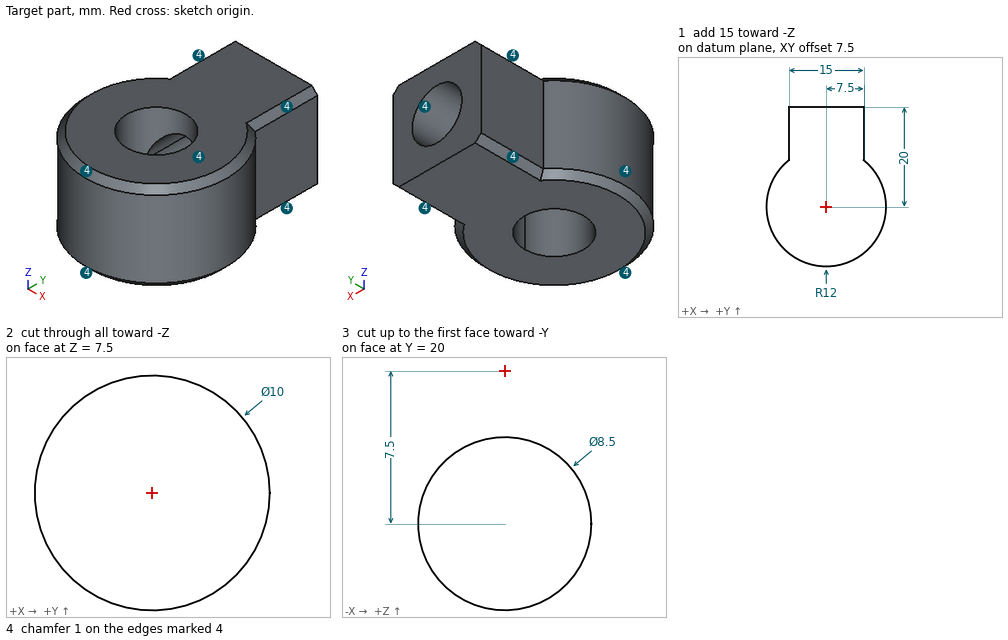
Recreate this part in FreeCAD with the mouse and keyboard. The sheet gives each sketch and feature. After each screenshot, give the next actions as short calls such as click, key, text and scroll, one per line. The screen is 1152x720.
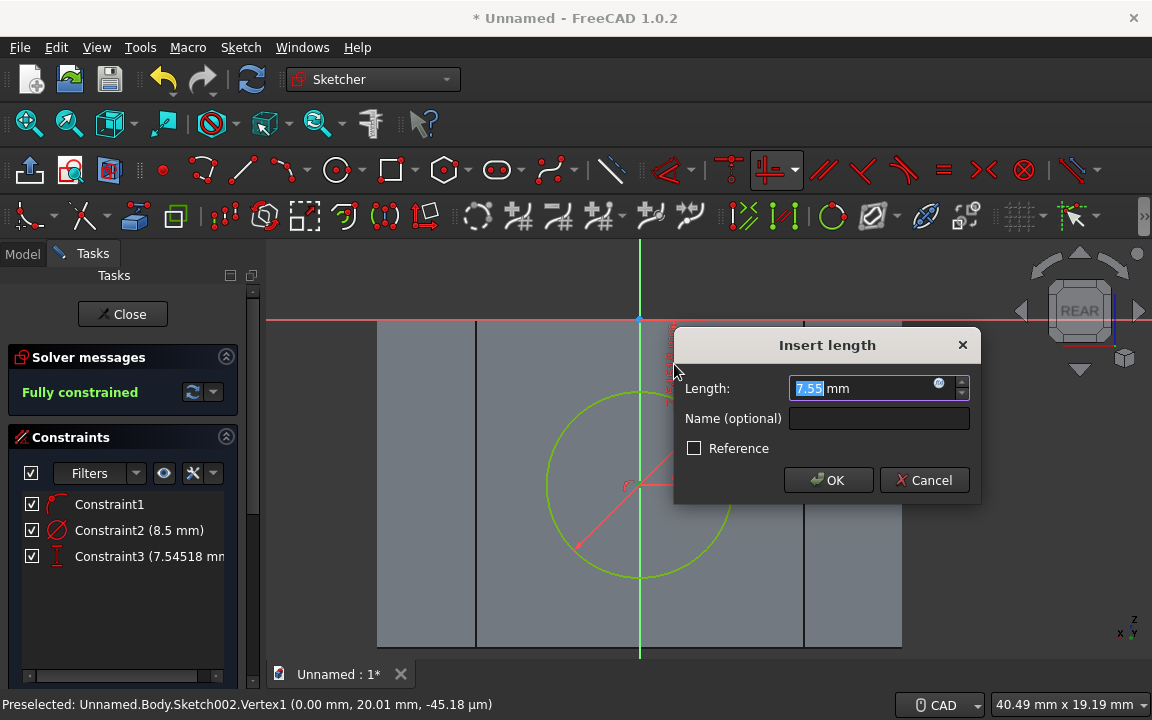
text(7.5)
key(Return)
key(Escape)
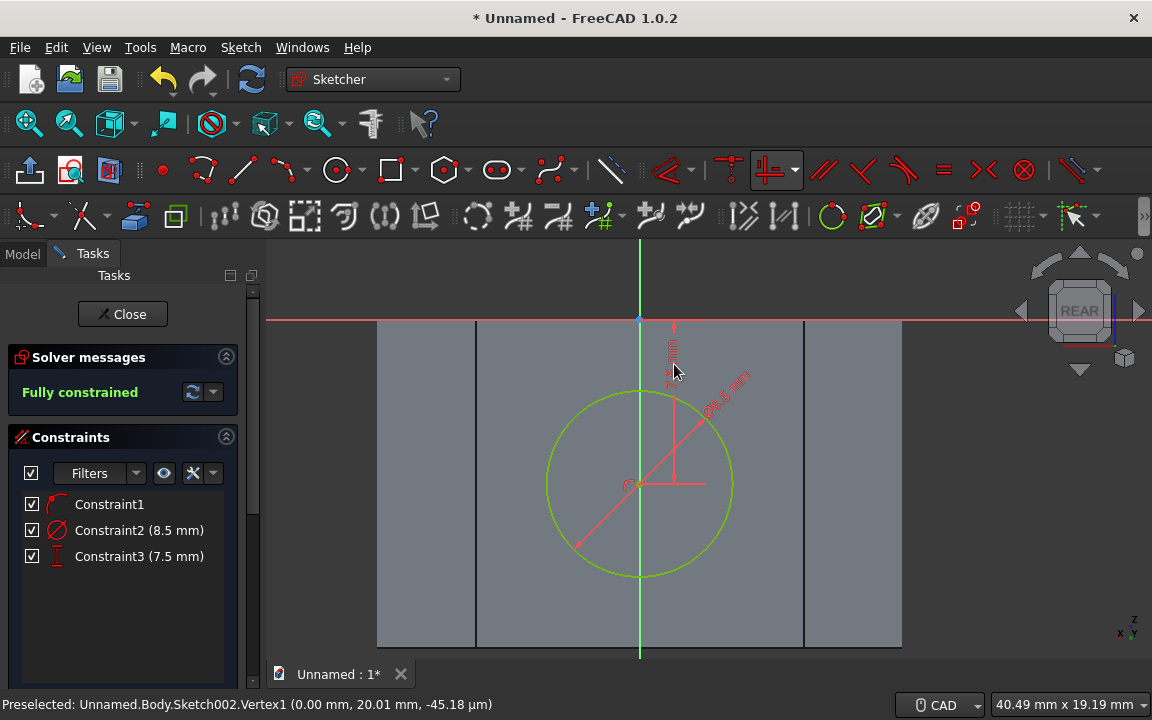
click(123, 314)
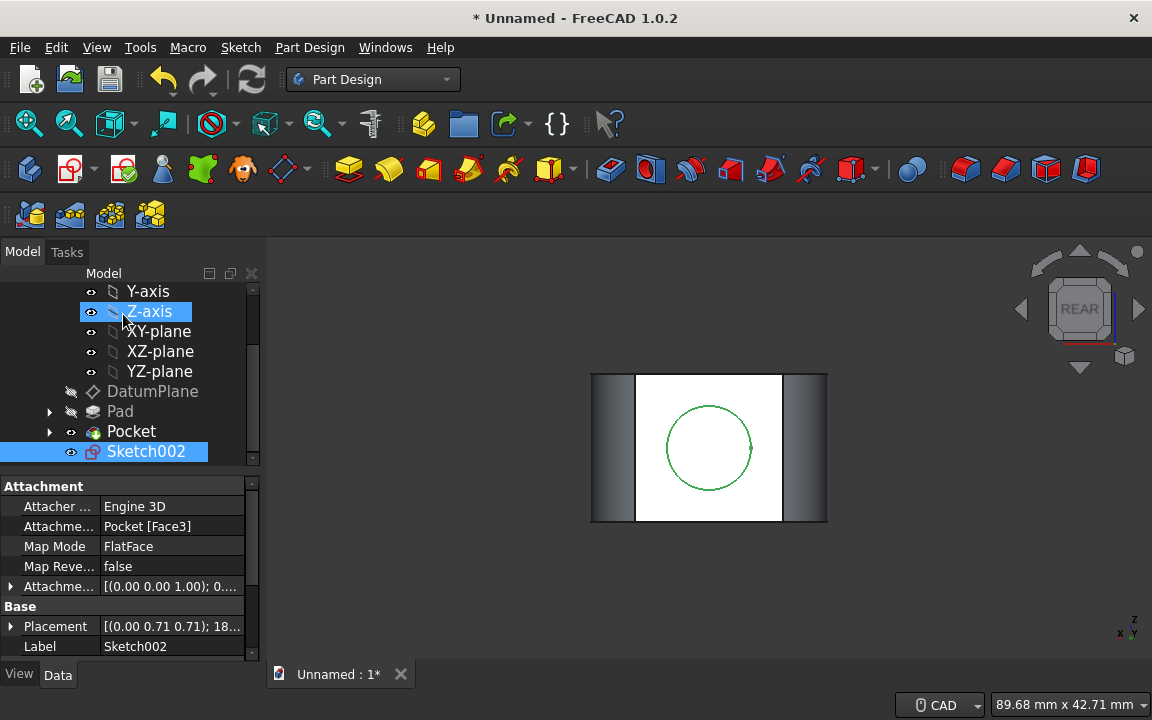
click(612, 170)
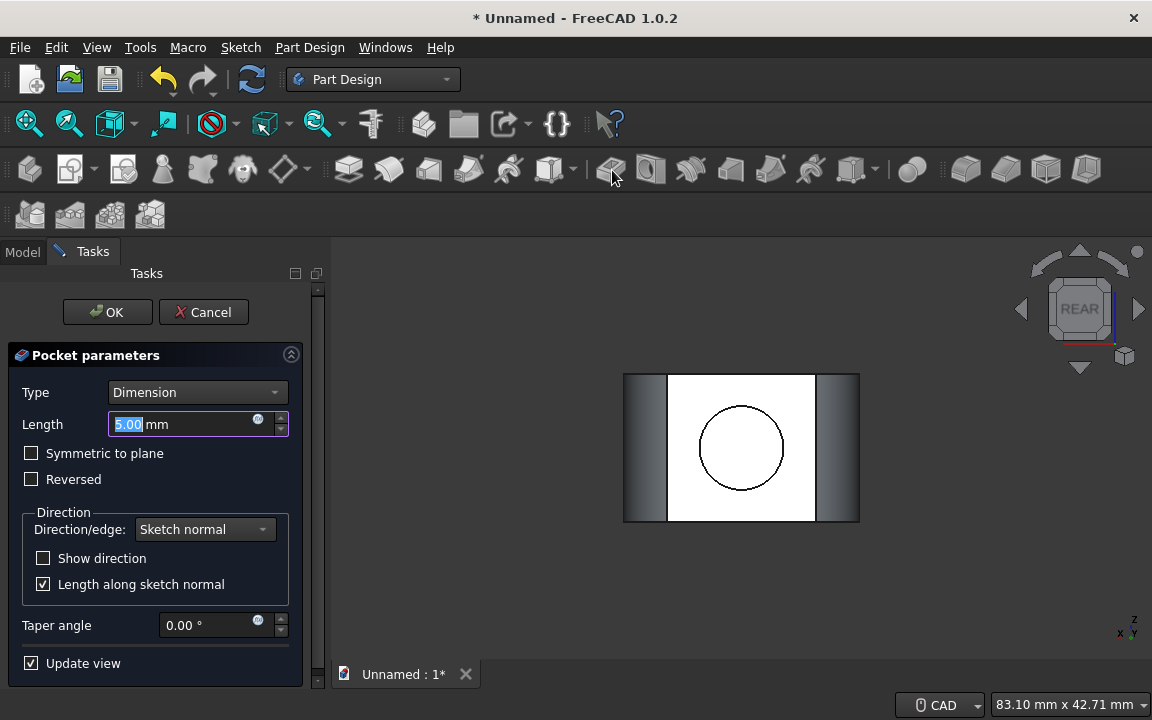
click(198, 392)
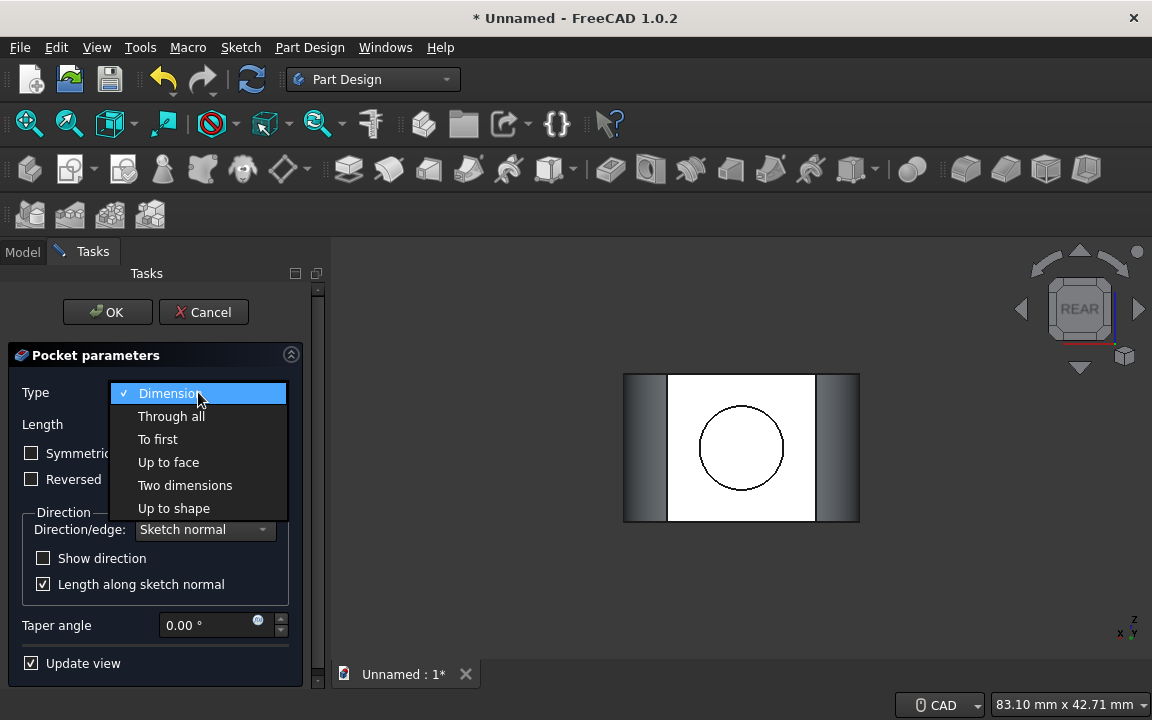
click(198, 440)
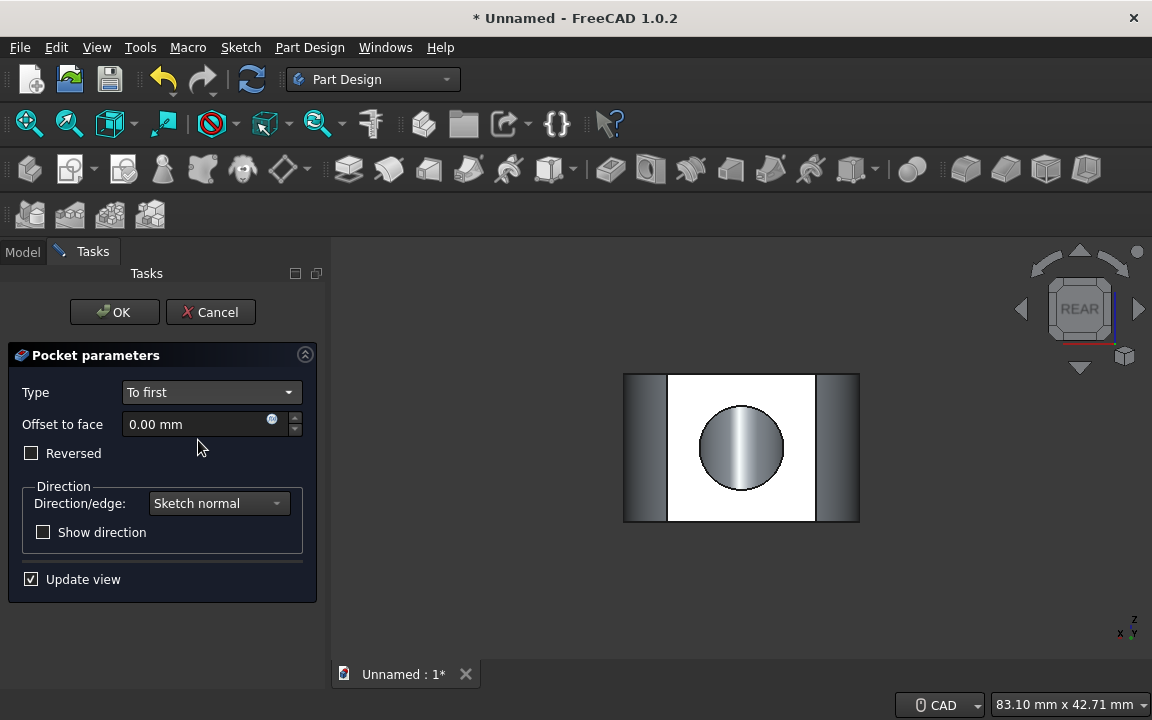
click(115, 312)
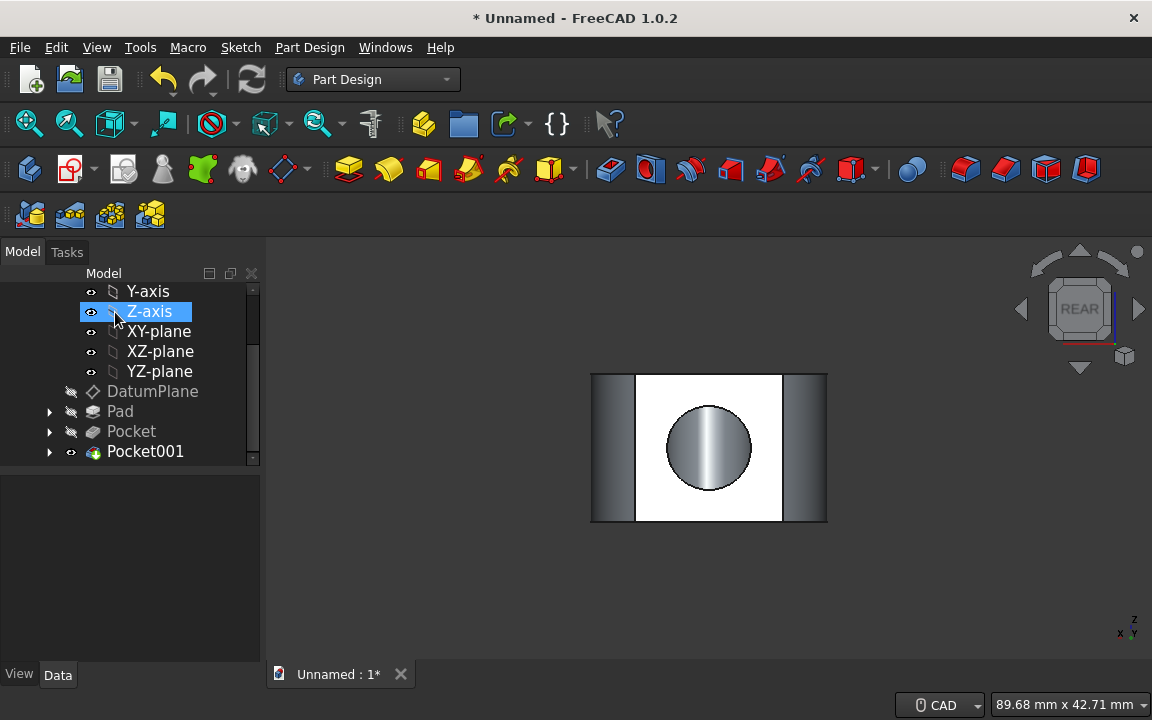
click(30, 124)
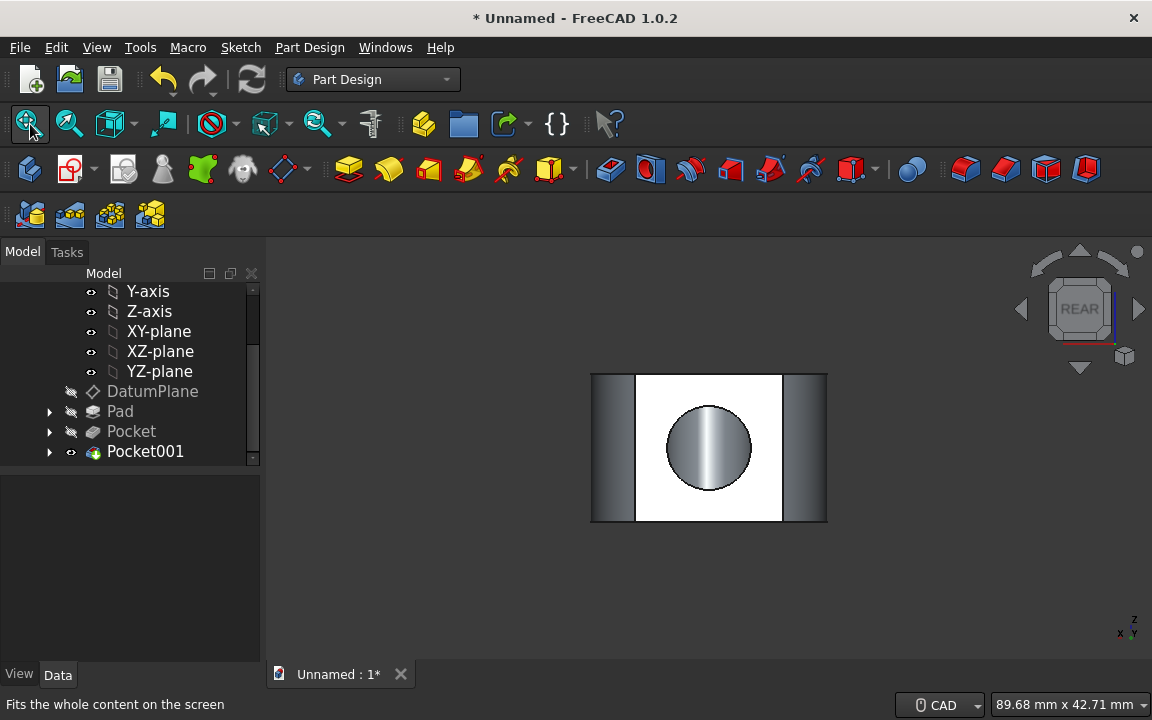
click(808, 521)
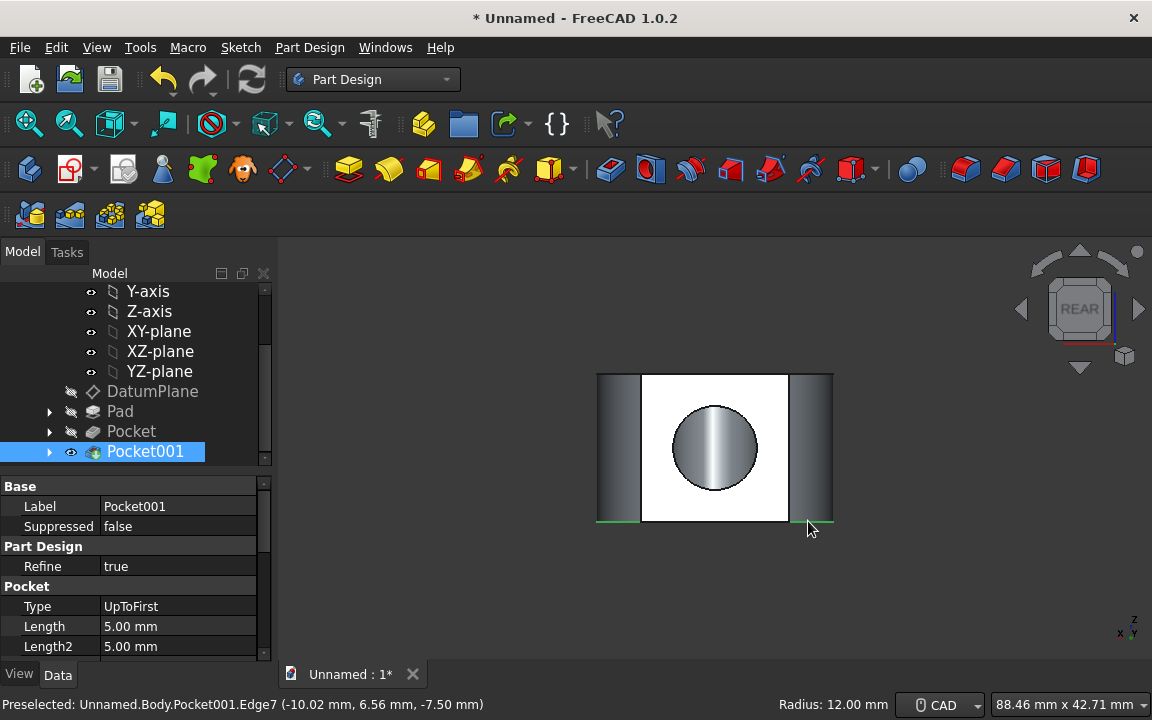
click(814, 373, ctrl)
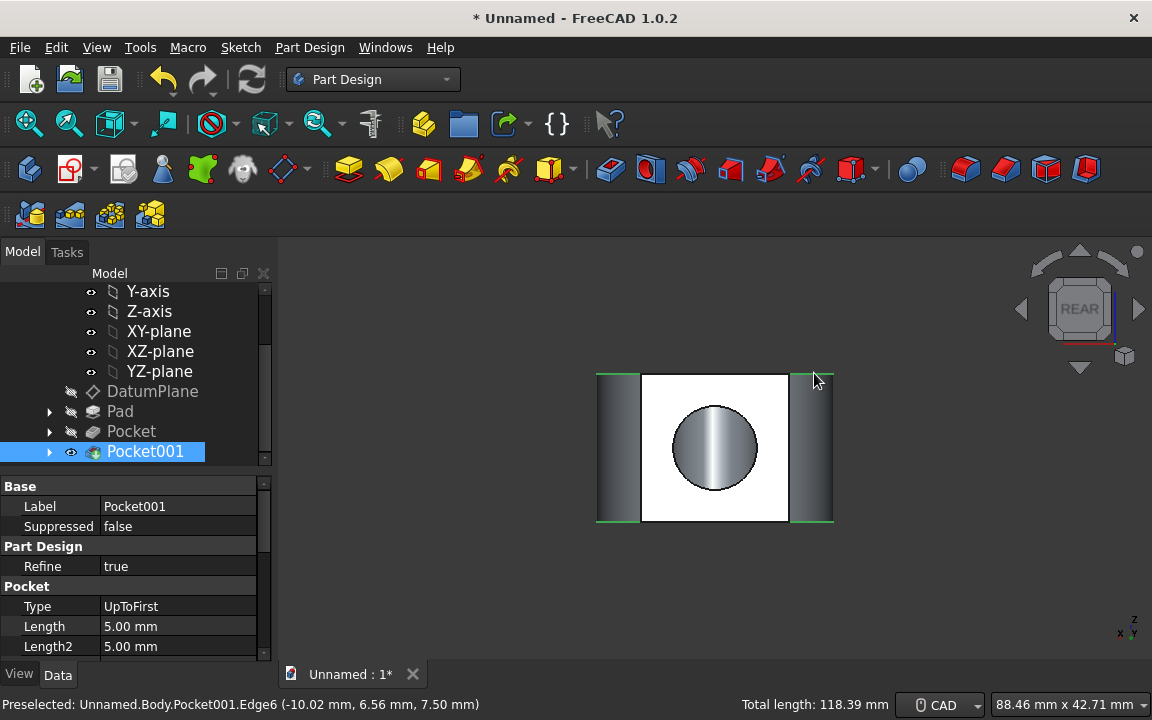
key(0)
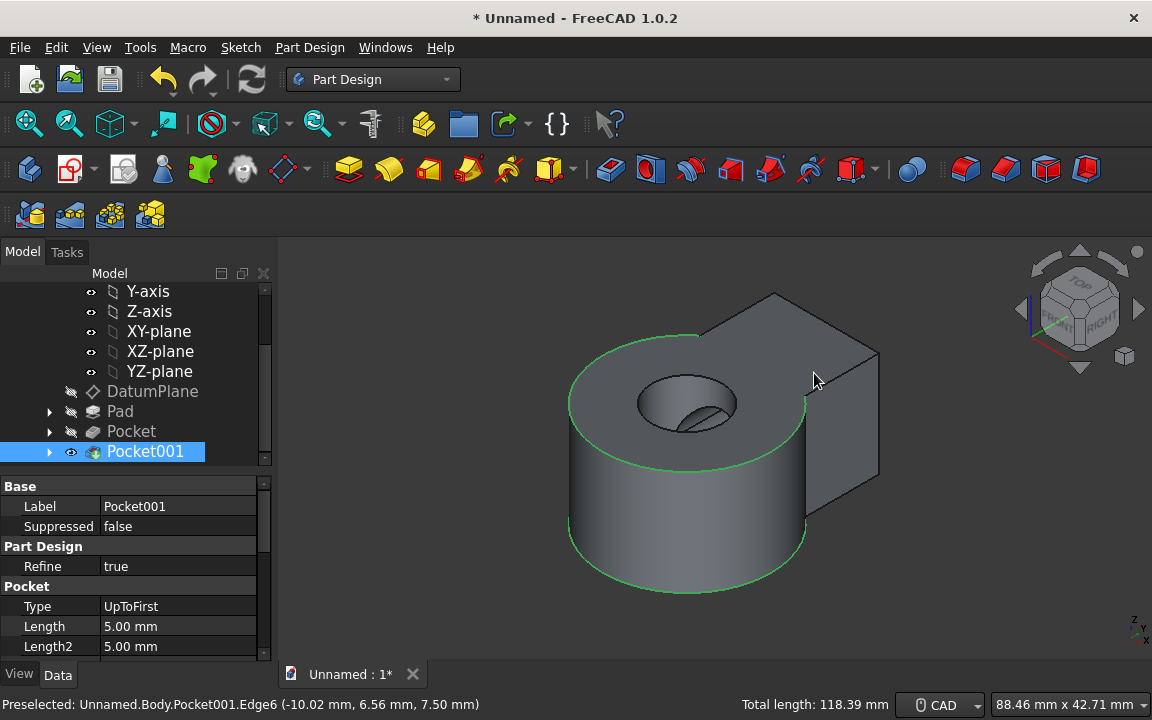
click(842, 374, ctrl)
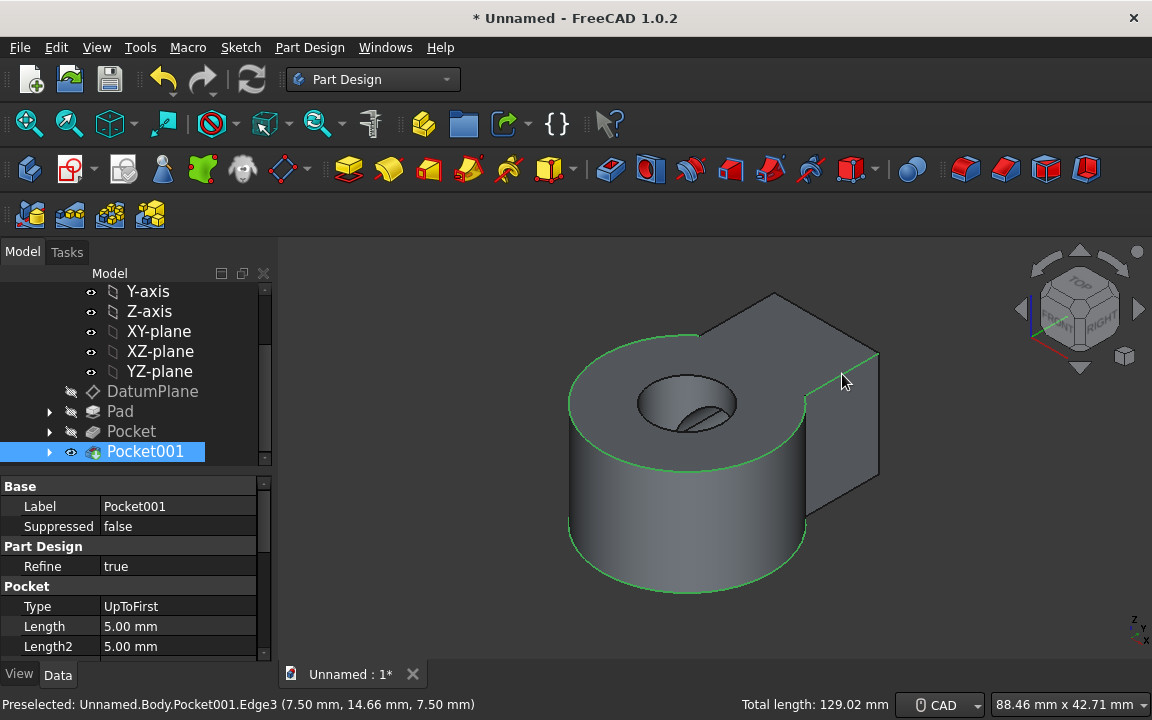
key(2)